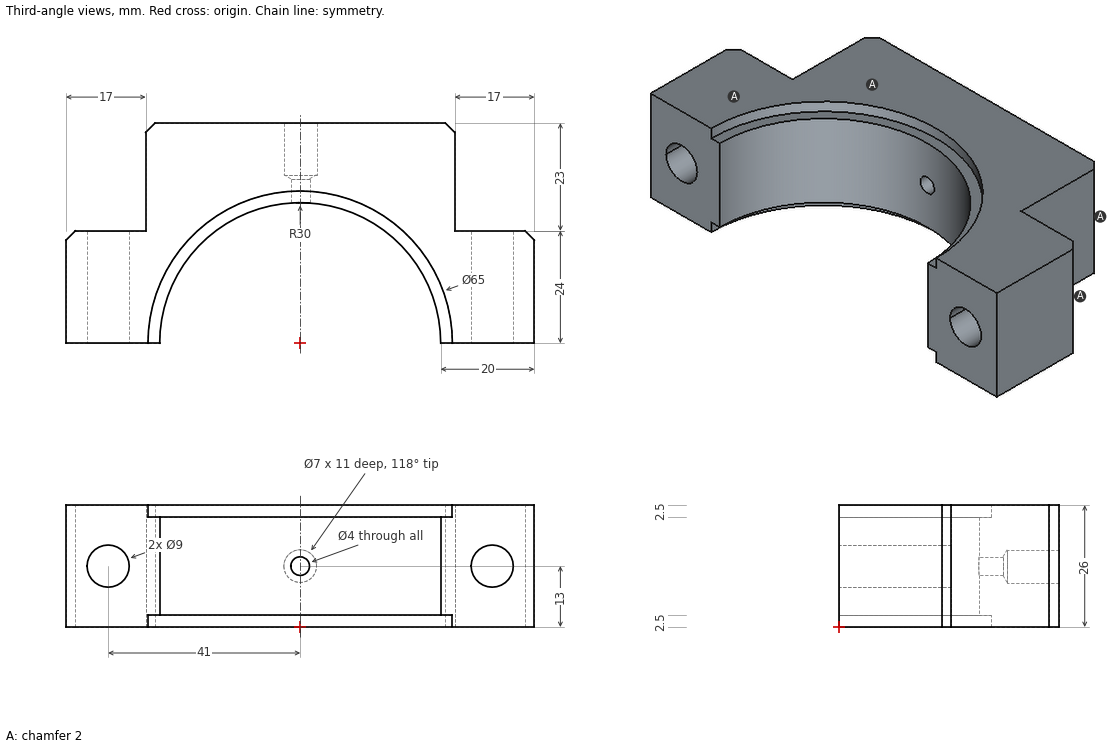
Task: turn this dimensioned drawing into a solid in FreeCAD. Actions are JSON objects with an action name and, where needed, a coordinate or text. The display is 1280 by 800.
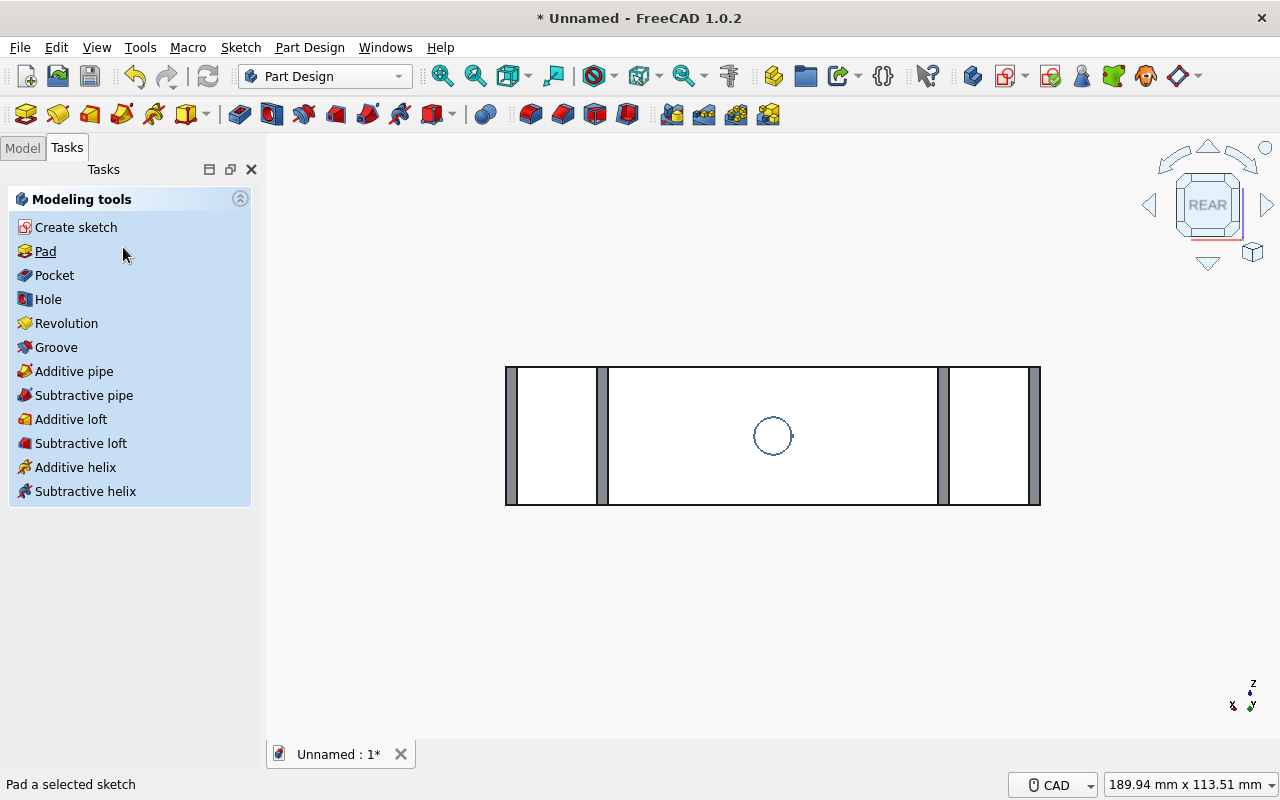
{"action": "left_click", "coordinate": [272, 114]}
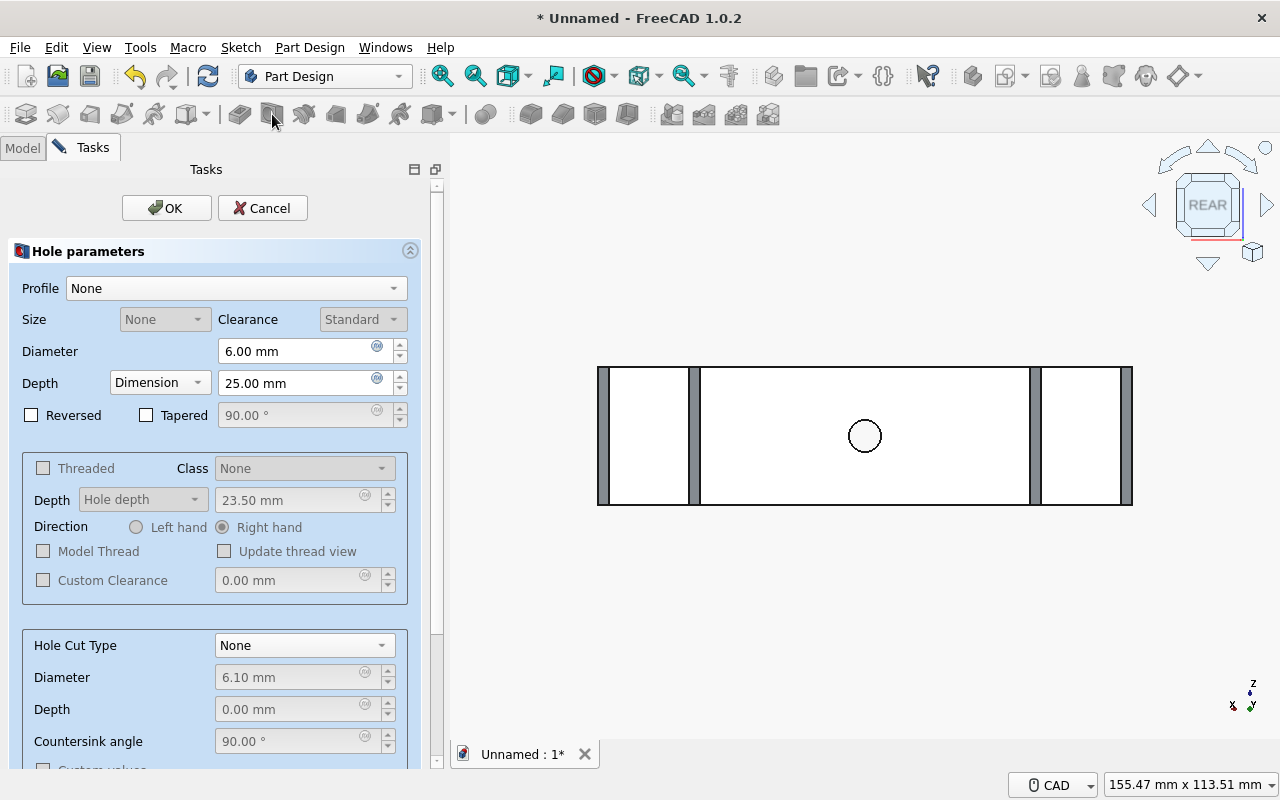
{"action": "triple_click", "coordinate": [305, 351]}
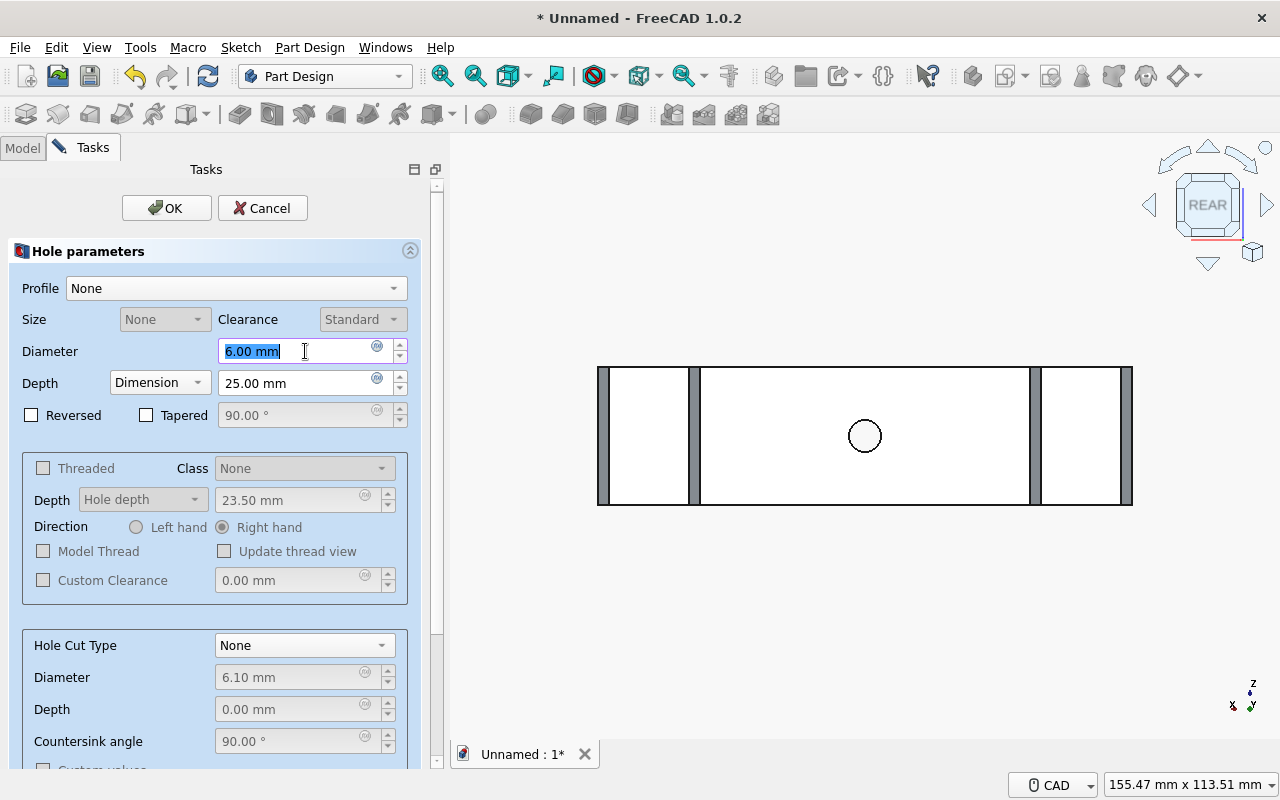
{"action": "type", "text": "7"}
{"action": "key", "text": "Tab"}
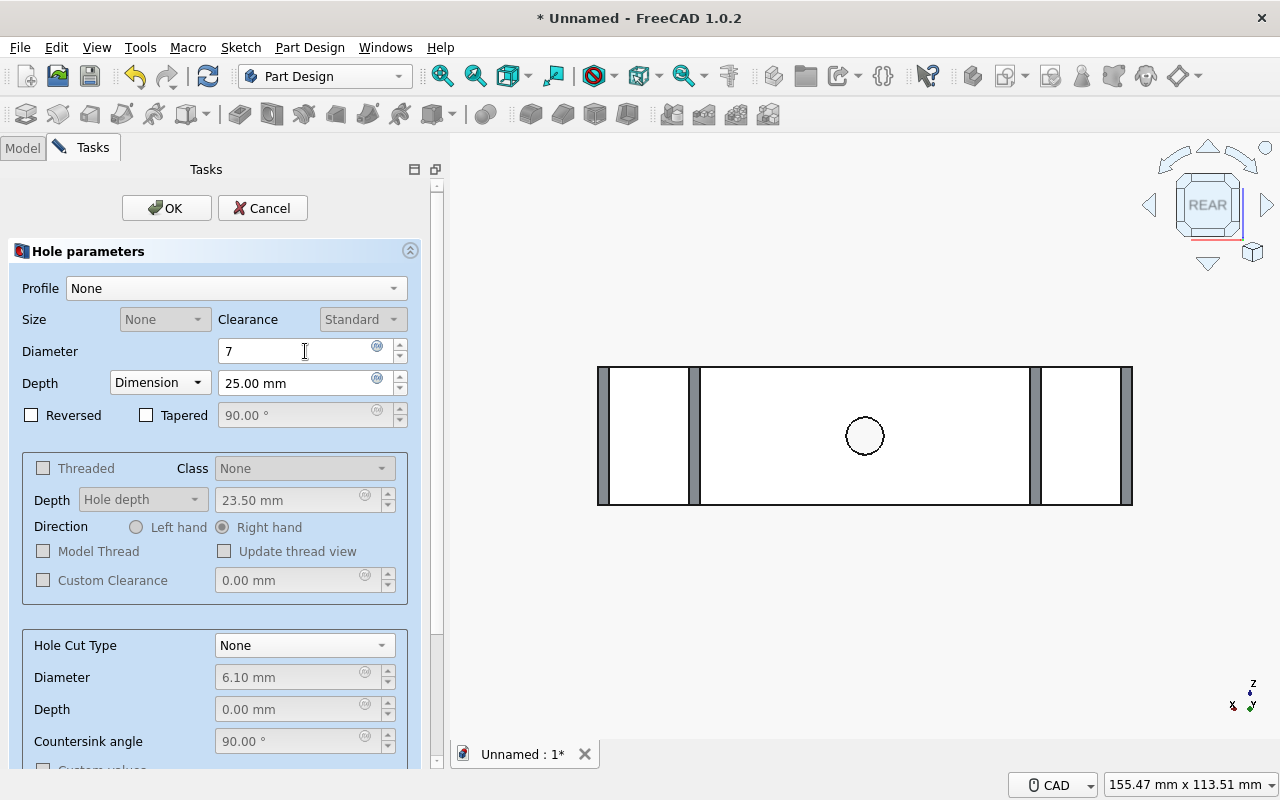
{"action": "triple_click", "coordinate": [305, 383]}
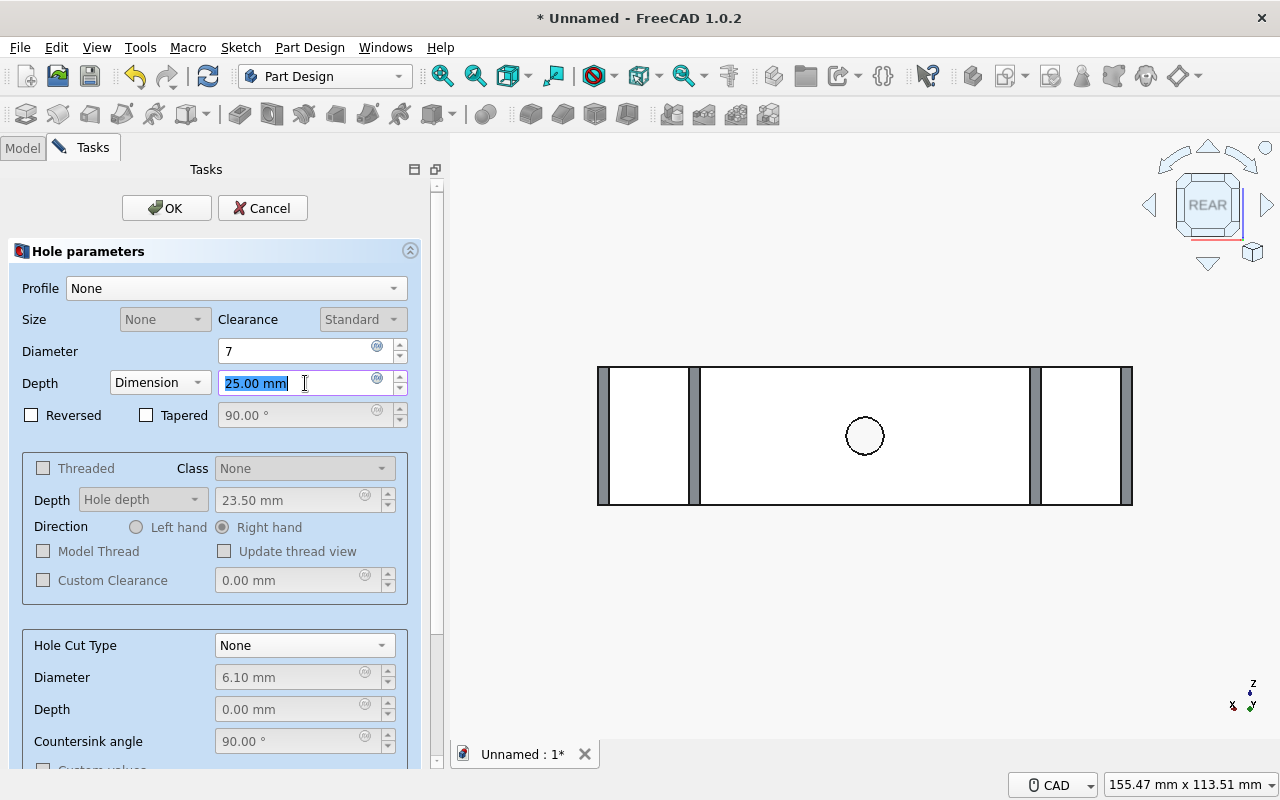
{"action": "type", "text": "11"}
{"action": "key", "text": "Tab"}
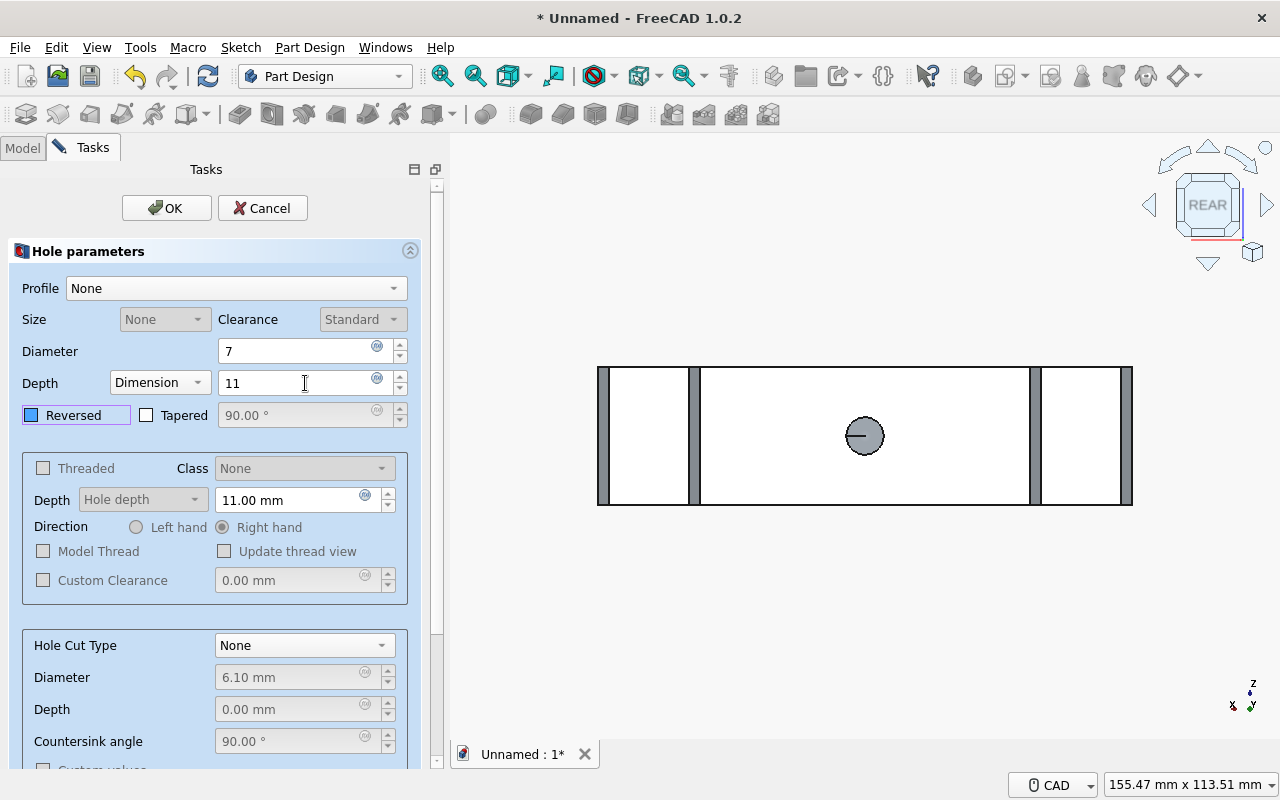
{"action": "left_click", "coordinate": [167, 208]}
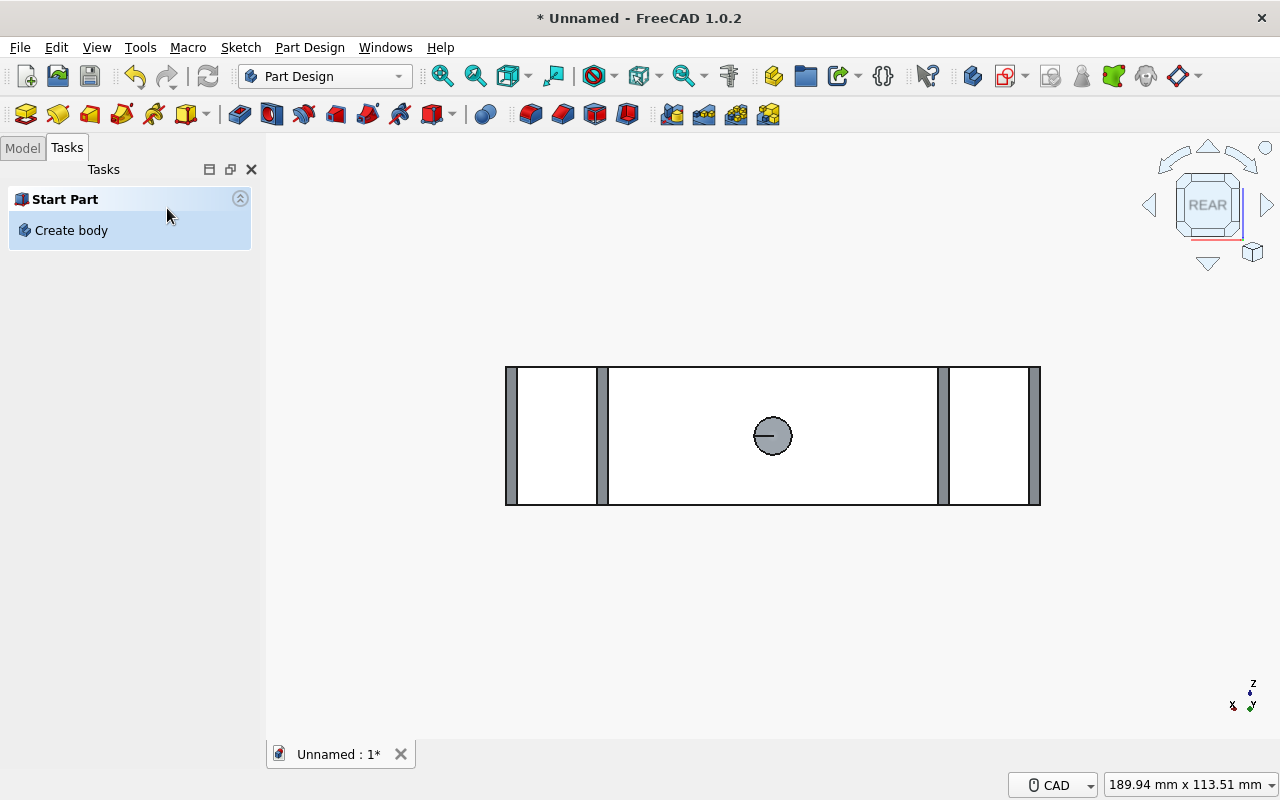
{"action": "left_click", "coordinate": [557, 415]}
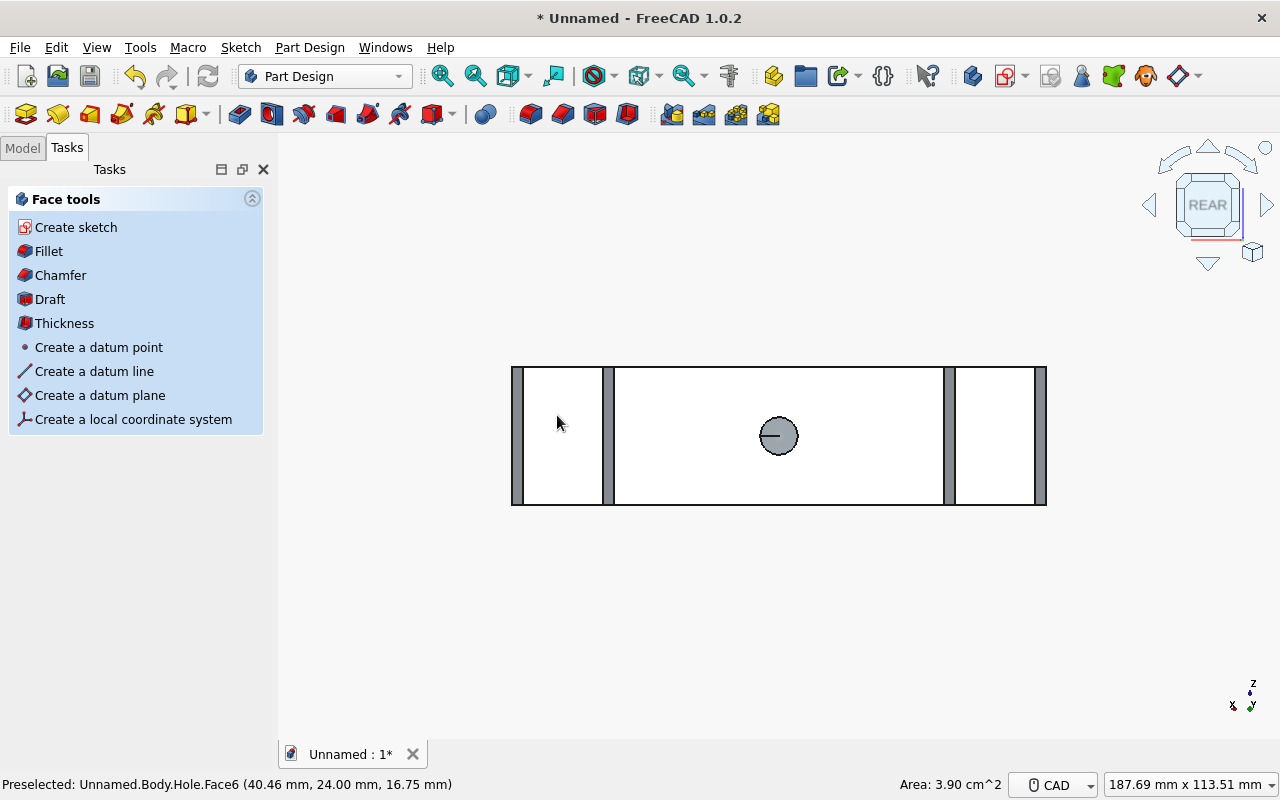
{"action": "left_click", "coordinate": [1006, 76]}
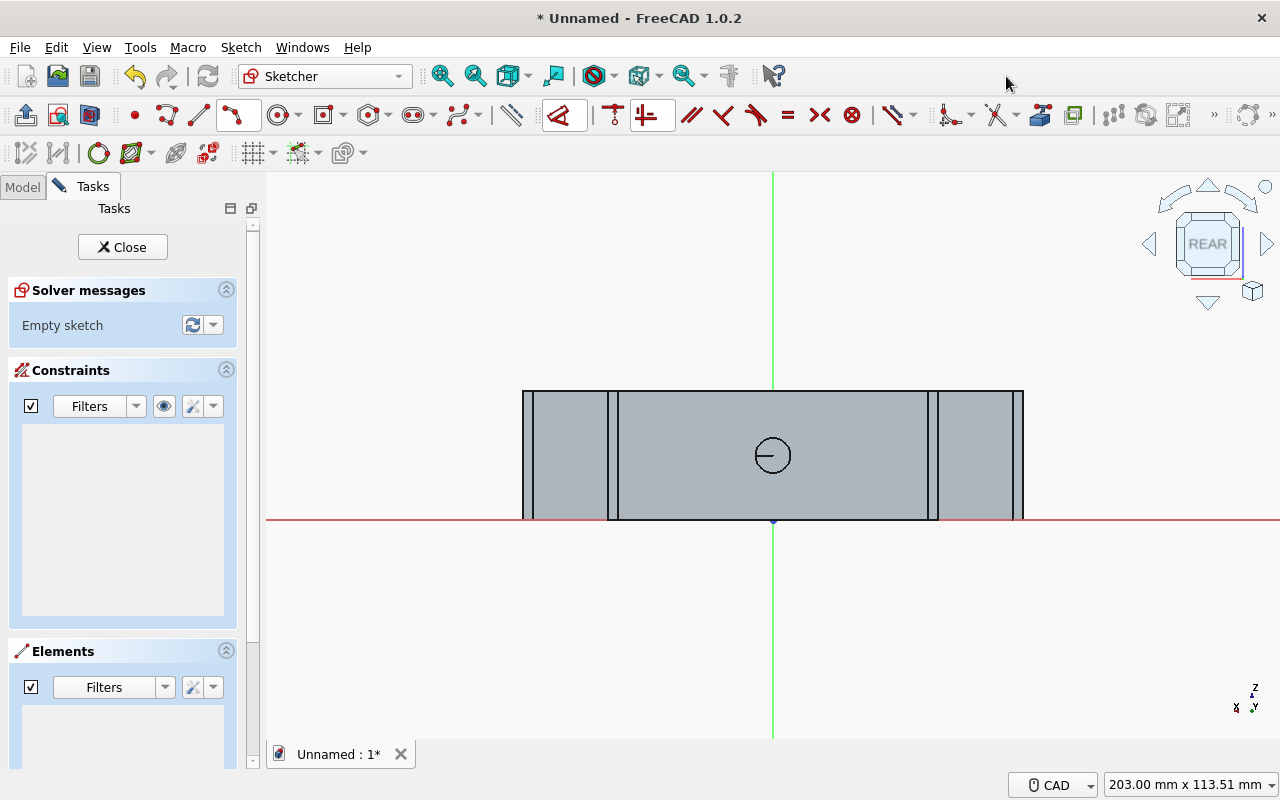
{"action": "key", "text": "g c"}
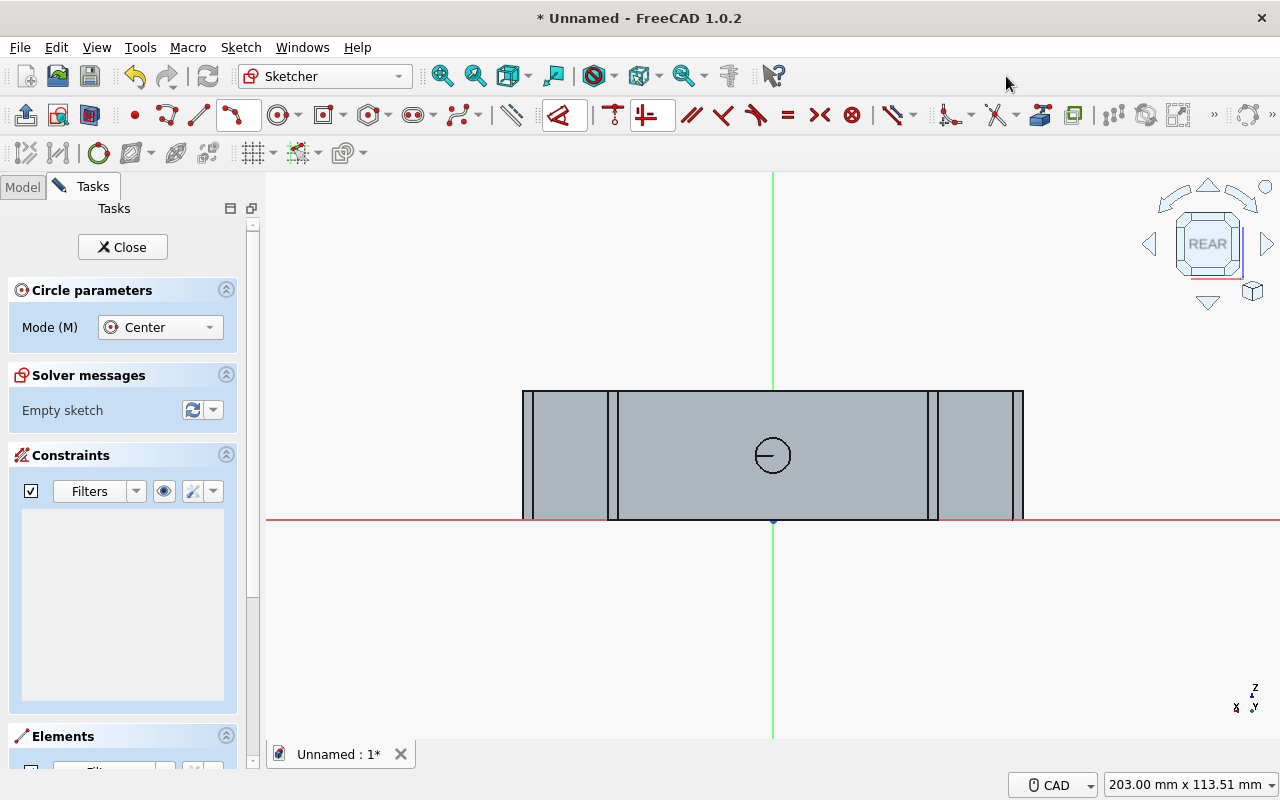
{"action": "left_click", "coordinate": [978, 456]}
{"action": "left_click", "coordinate": [994, 440]}